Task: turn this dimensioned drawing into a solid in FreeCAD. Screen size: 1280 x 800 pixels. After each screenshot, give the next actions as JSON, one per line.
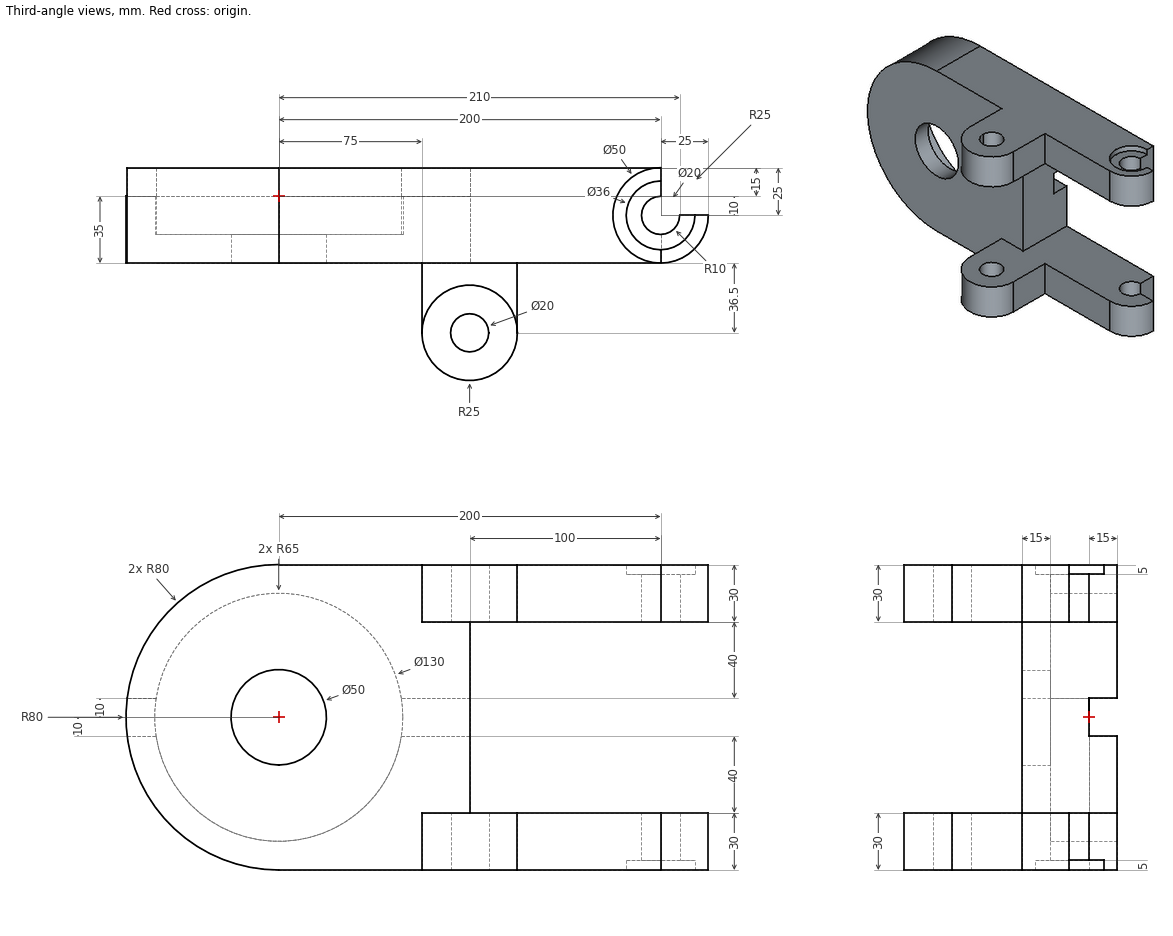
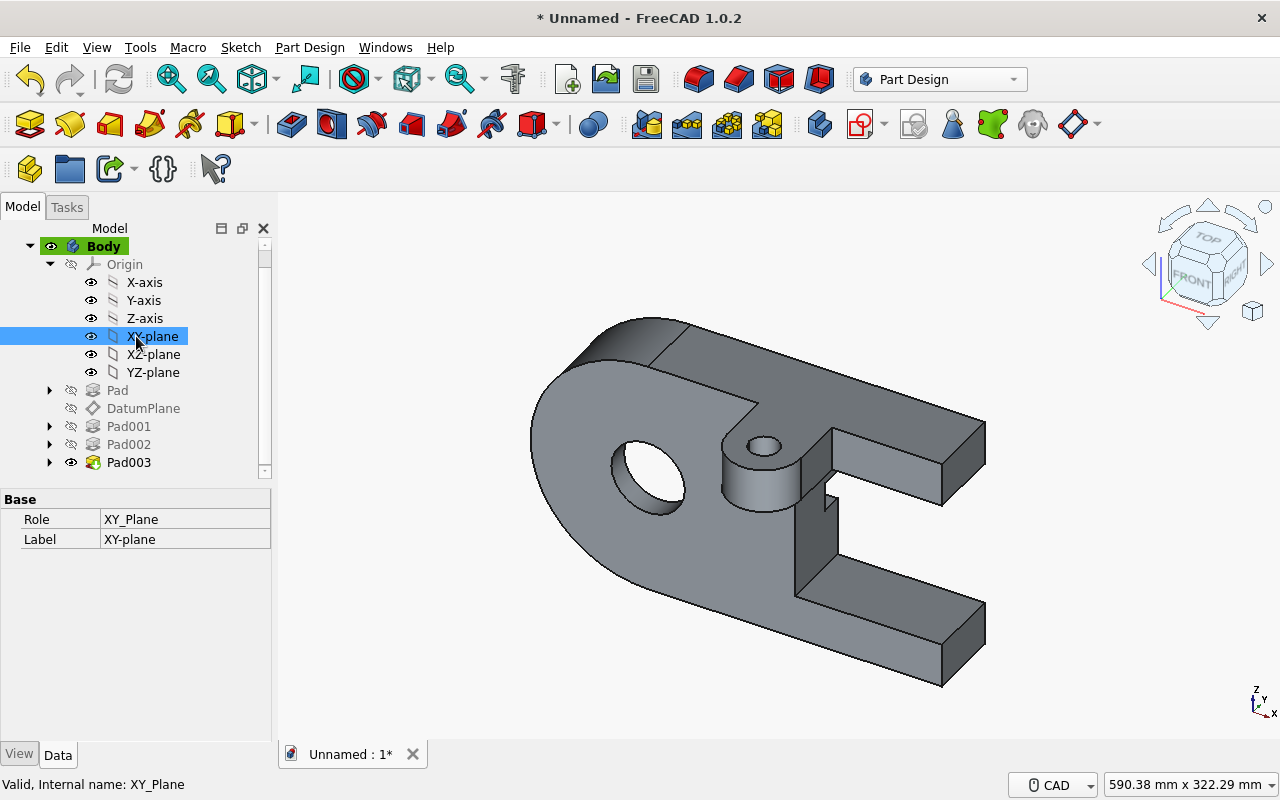
{"action": "left_click", "coordinate": [1074, 124]}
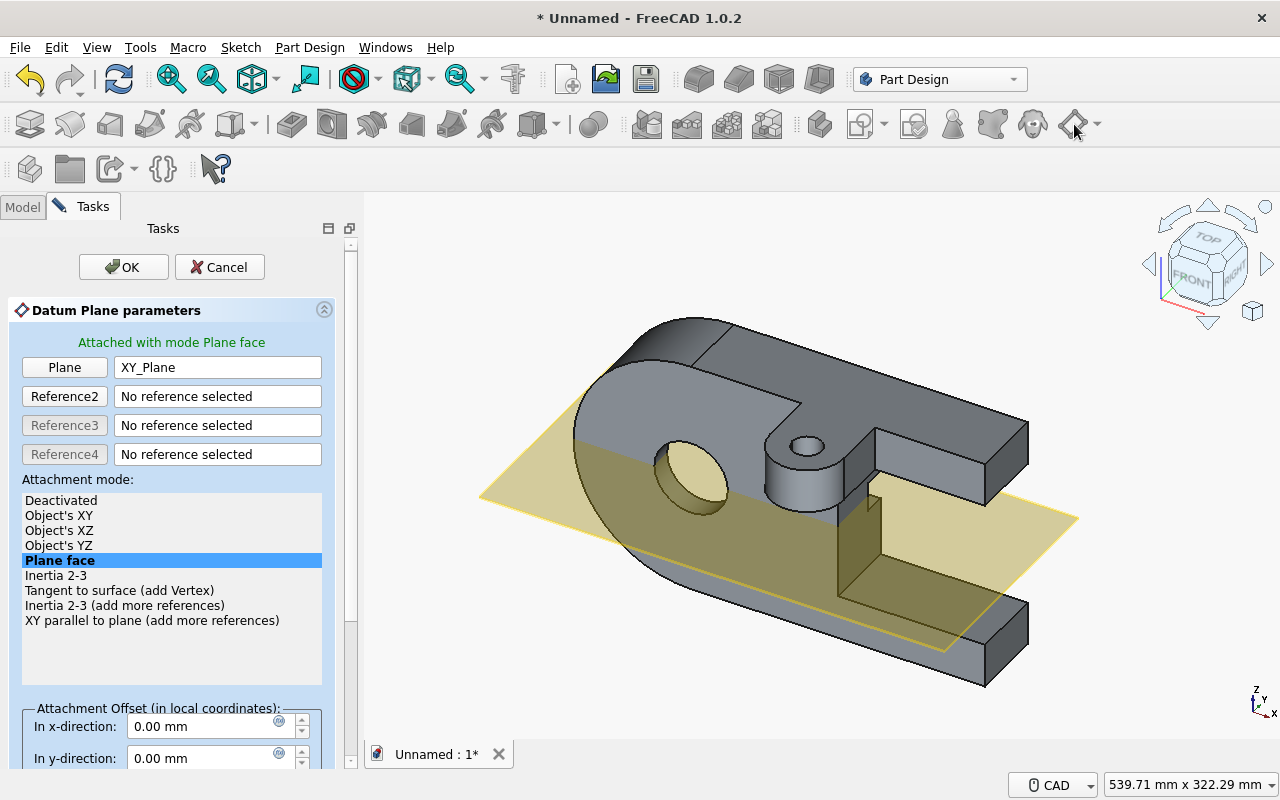
{"action": "scroll", "coordinate": [351, 503], "scroll_direction": "down", "scroll_amount": 2}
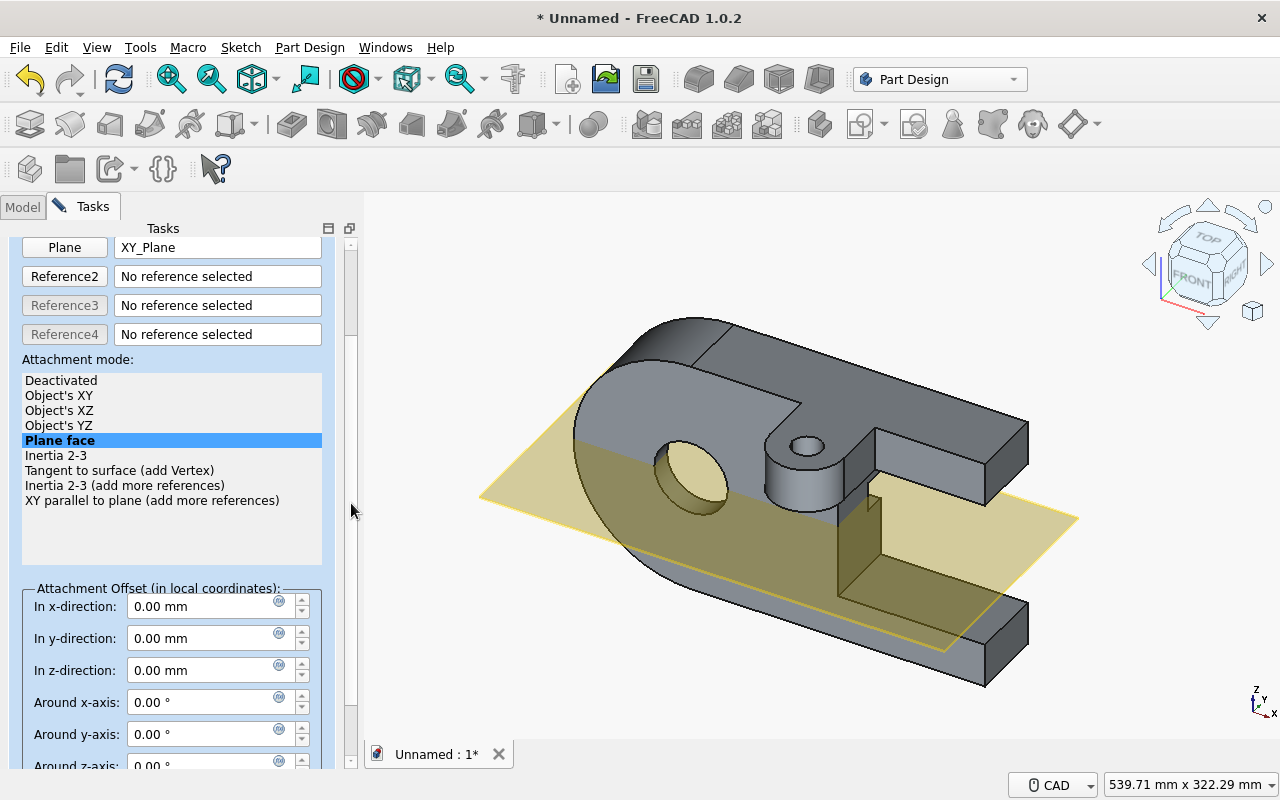
{"action": "triple_click", "coordinate": [210, 670]}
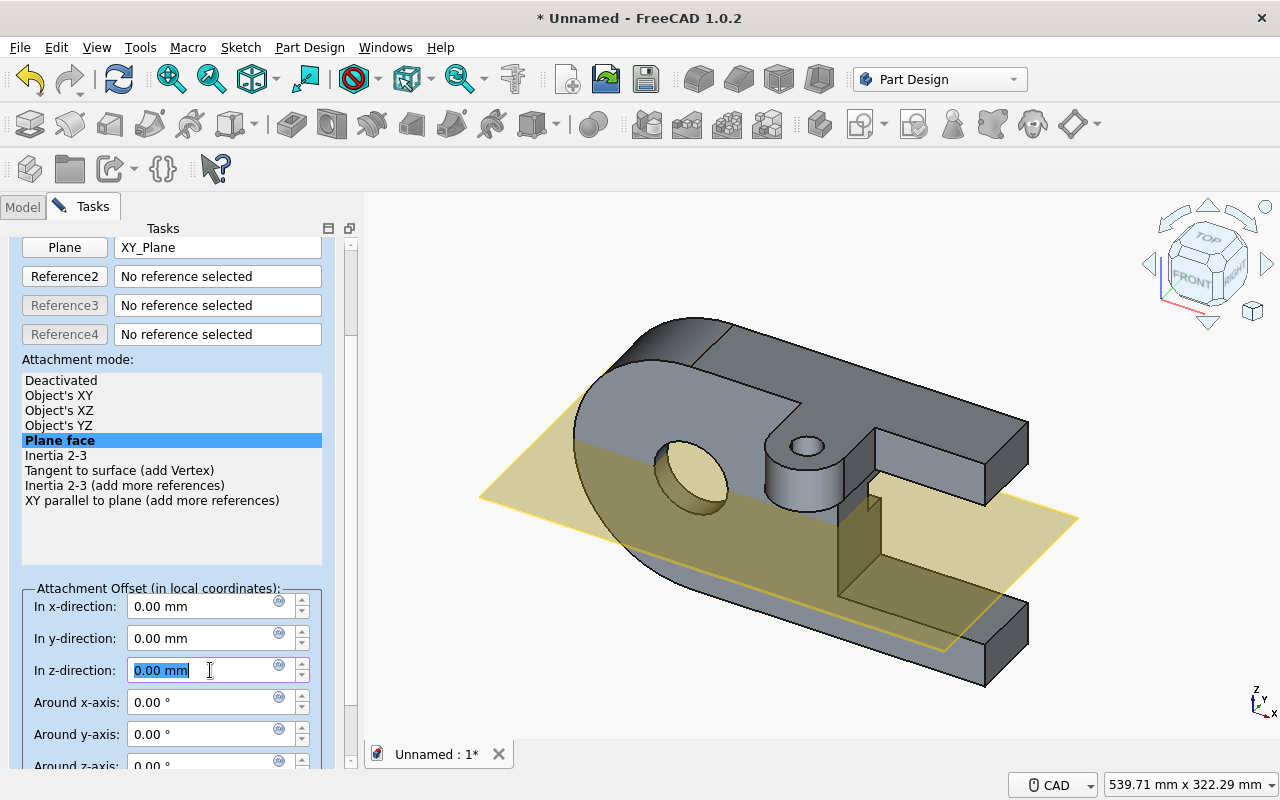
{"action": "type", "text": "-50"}
{"action": "key", "text": "Tab"}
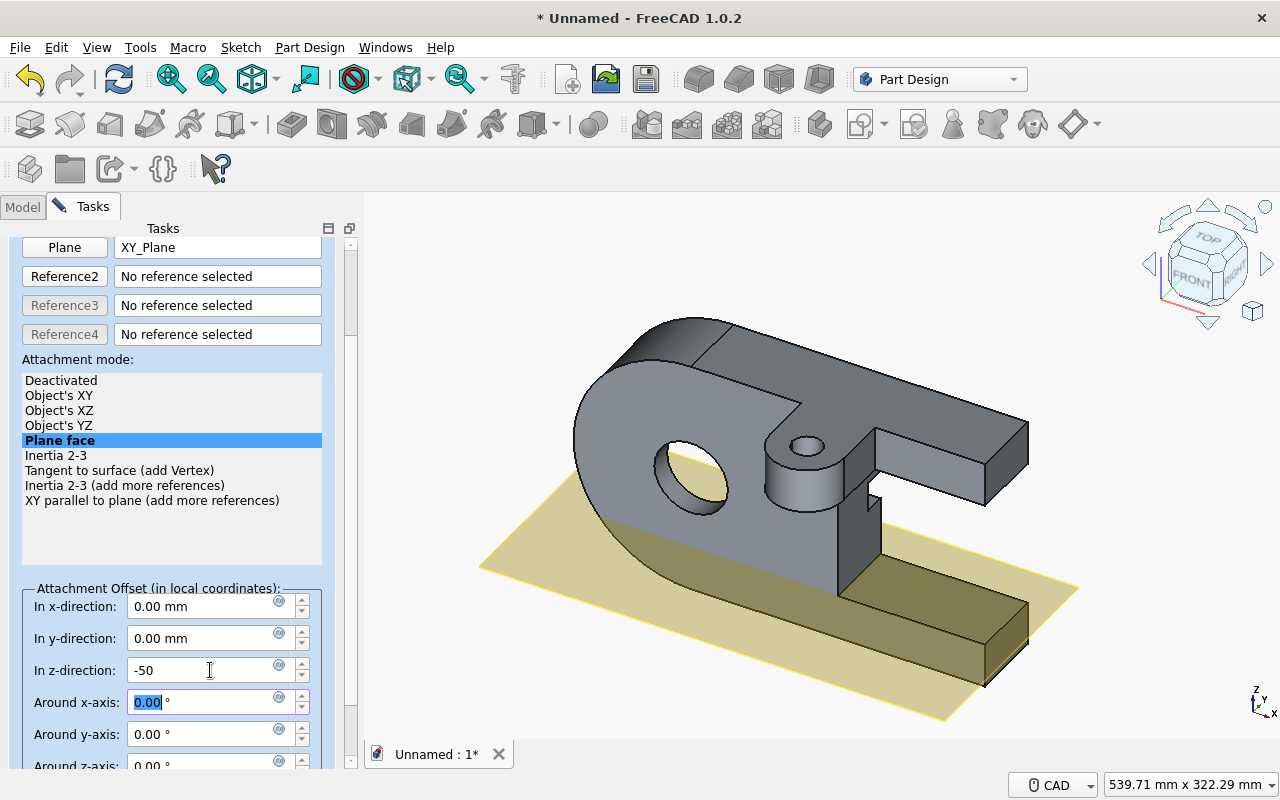
{"action": "scroll", "coordinate": [351, 503], "scroll_direction": "up", "scroll_amount": 3}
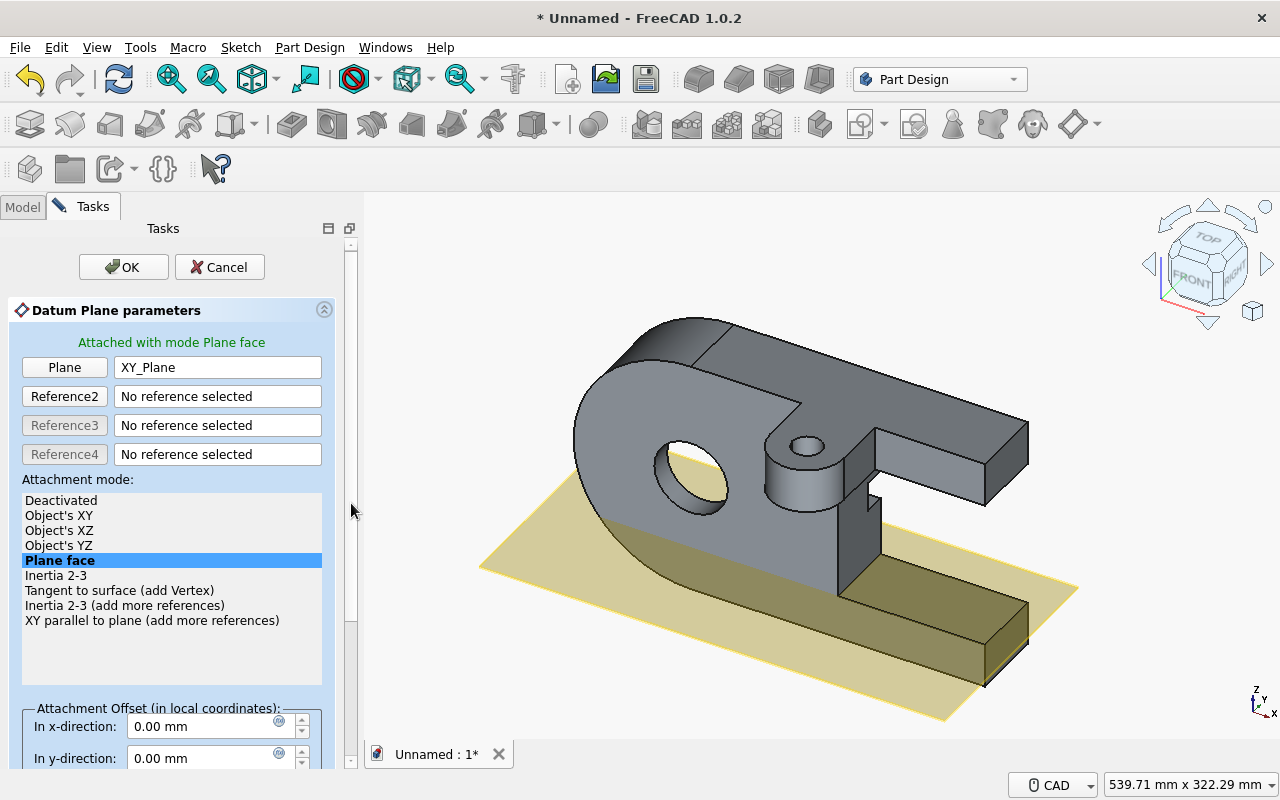
{"action": "left_click", "coordinate": [124, 267]}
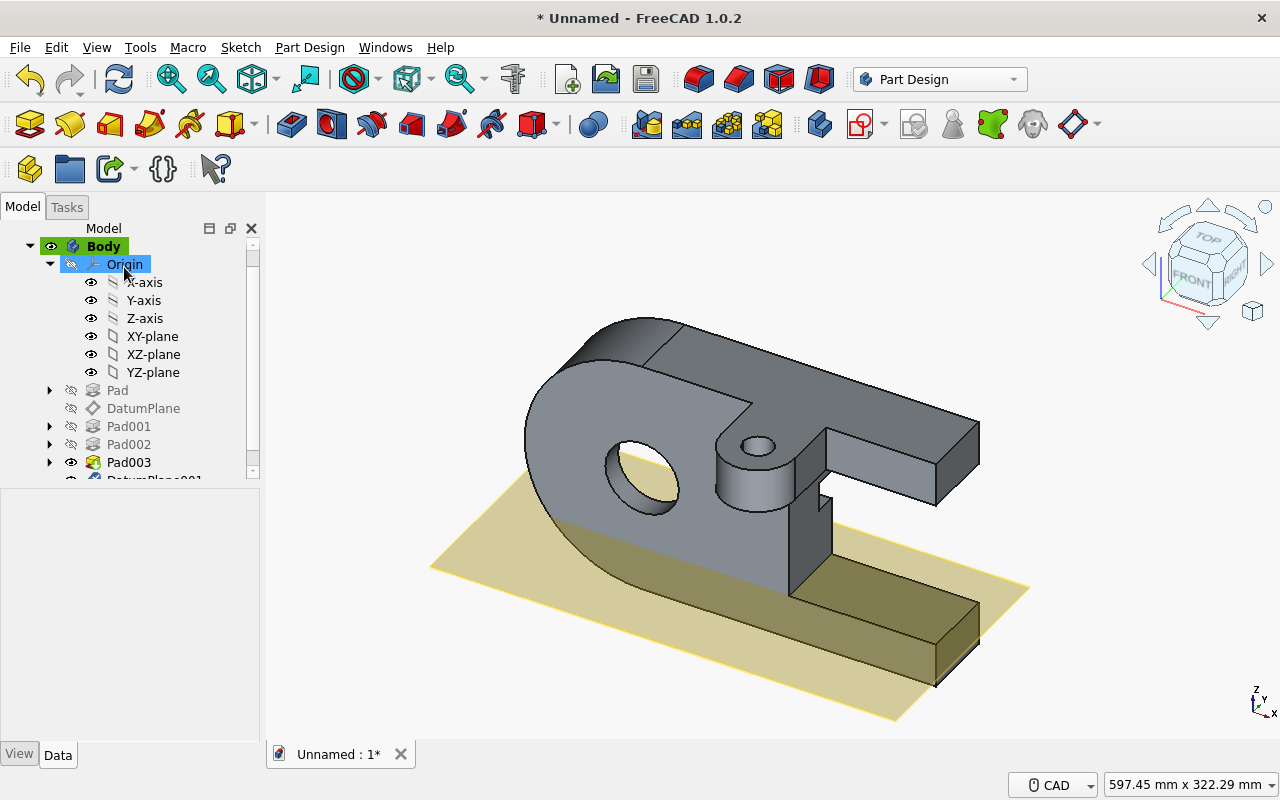
{"action": "scroll", "coordinate": [120, 350], "scroll_direction": "down", "scroll_amount": 3}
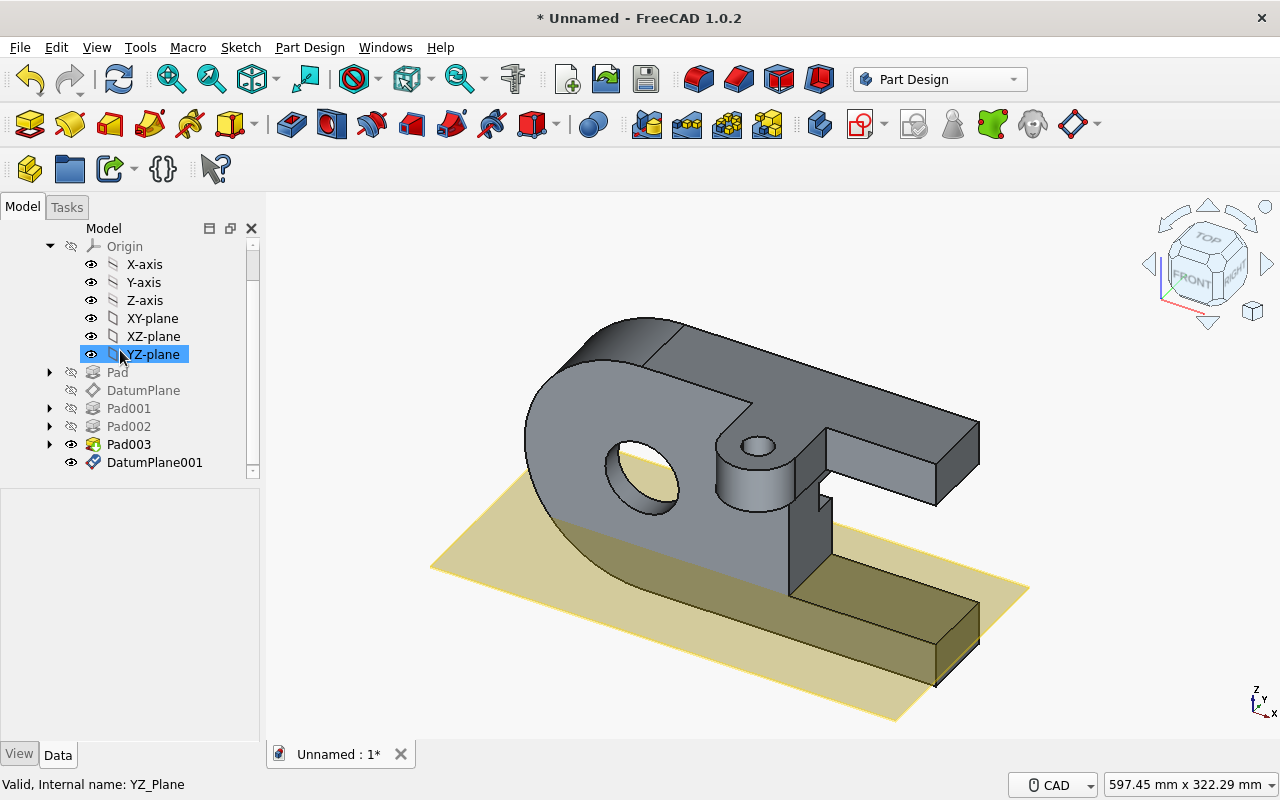
{"action": "left_click", "coordinate": [116, 462]}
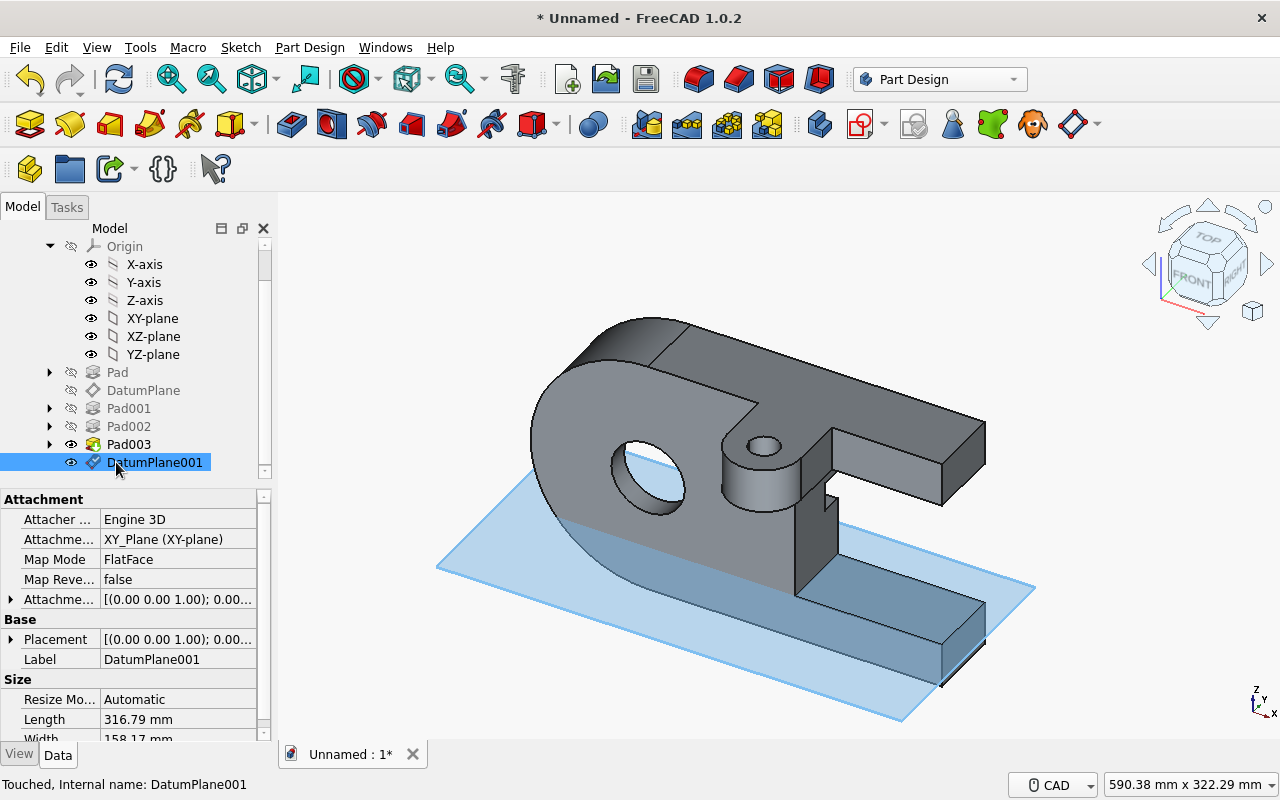
{"action": "left_click", "coordinate": [860, 124]}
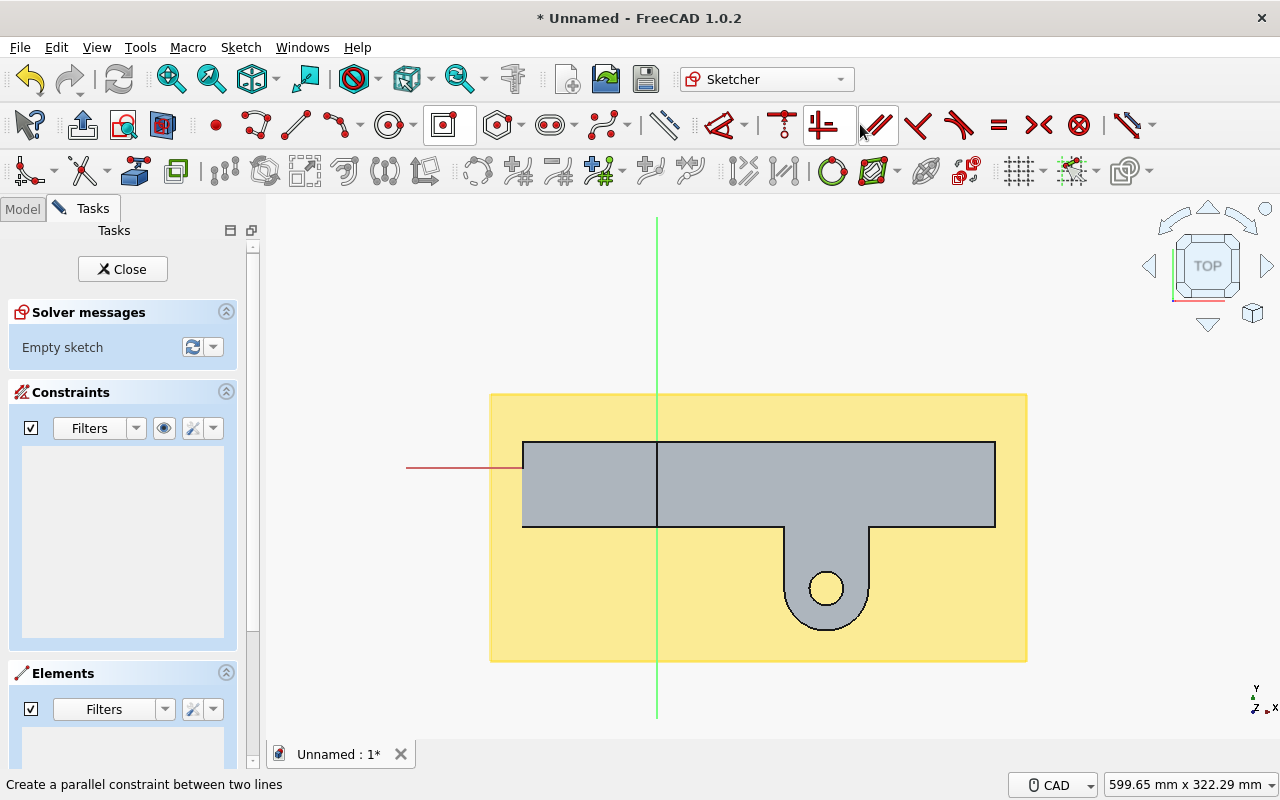
{"action": "key", "text": "q s"}